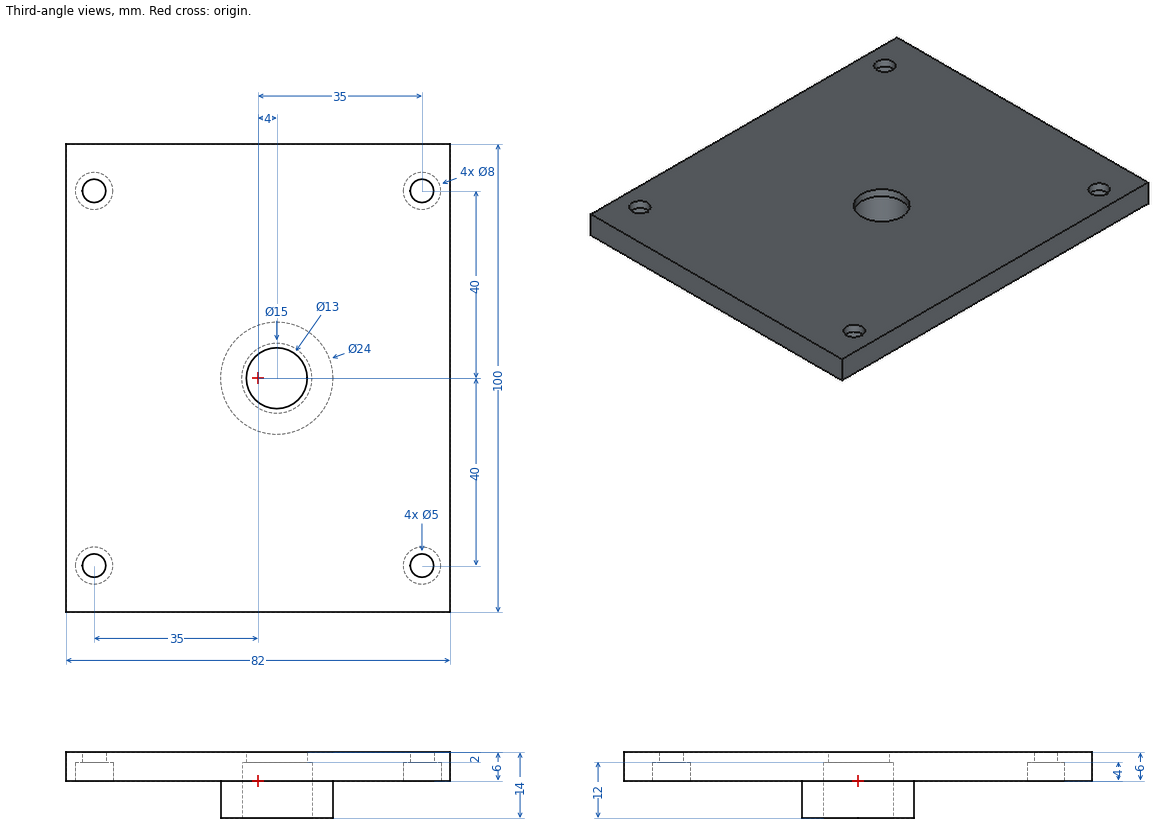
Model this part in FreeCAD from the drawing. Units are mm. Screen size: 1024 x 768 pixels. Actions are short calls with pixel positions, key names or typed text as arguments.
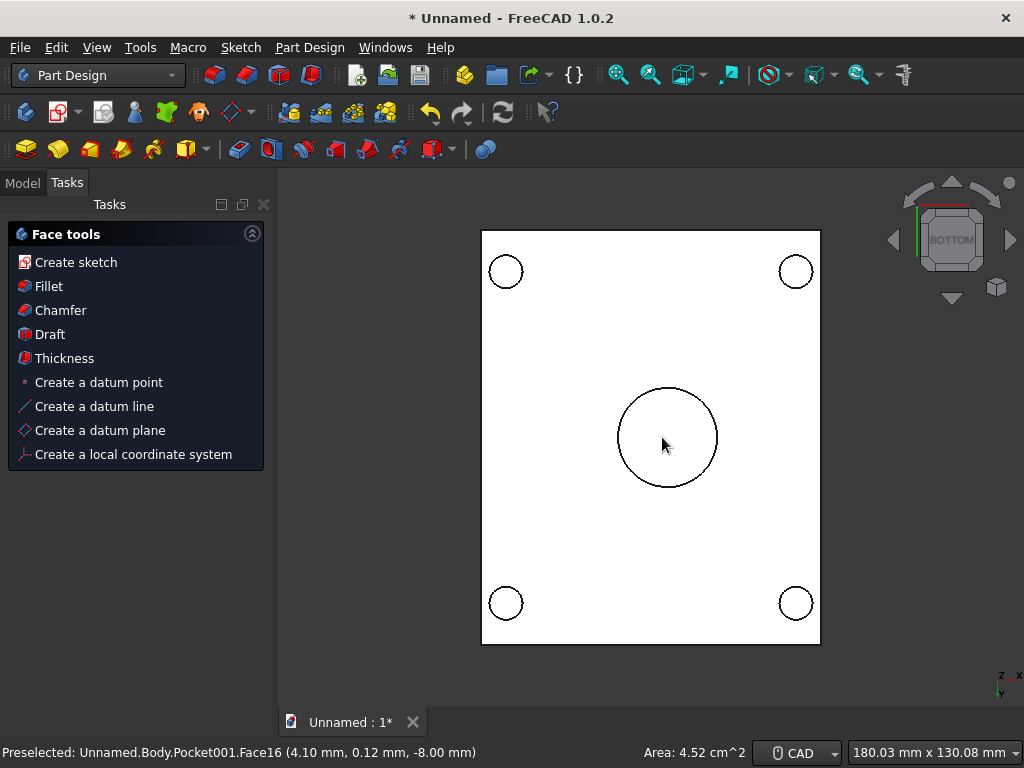
click(58, 112)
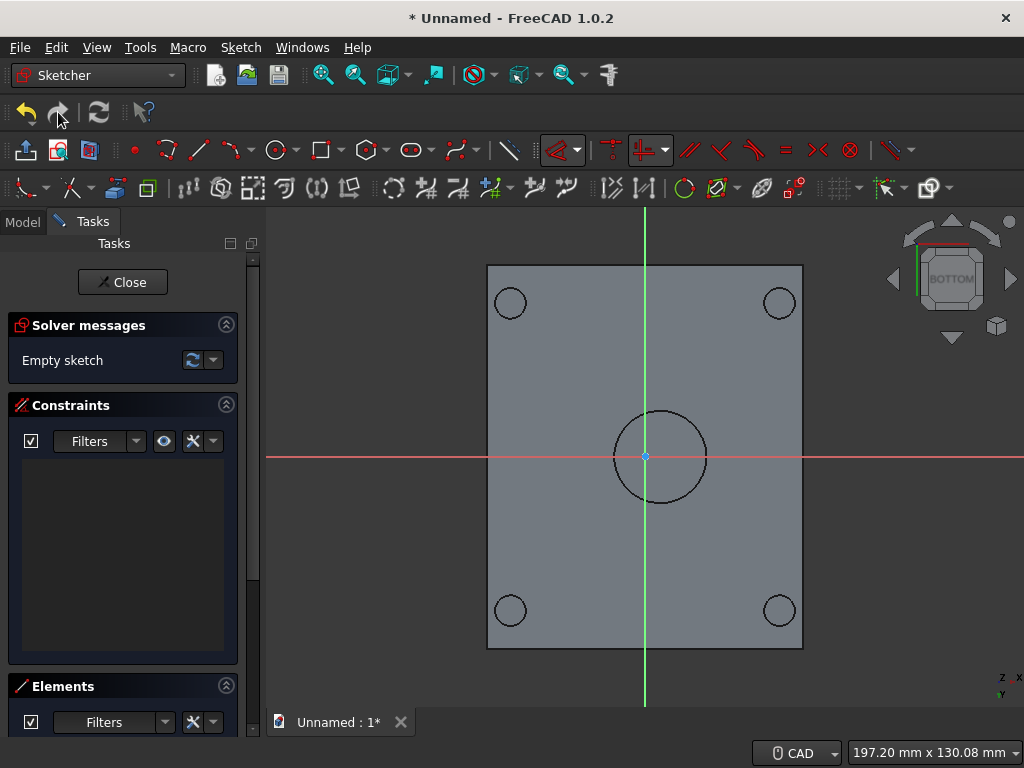
scroll(682, 457, up, 8)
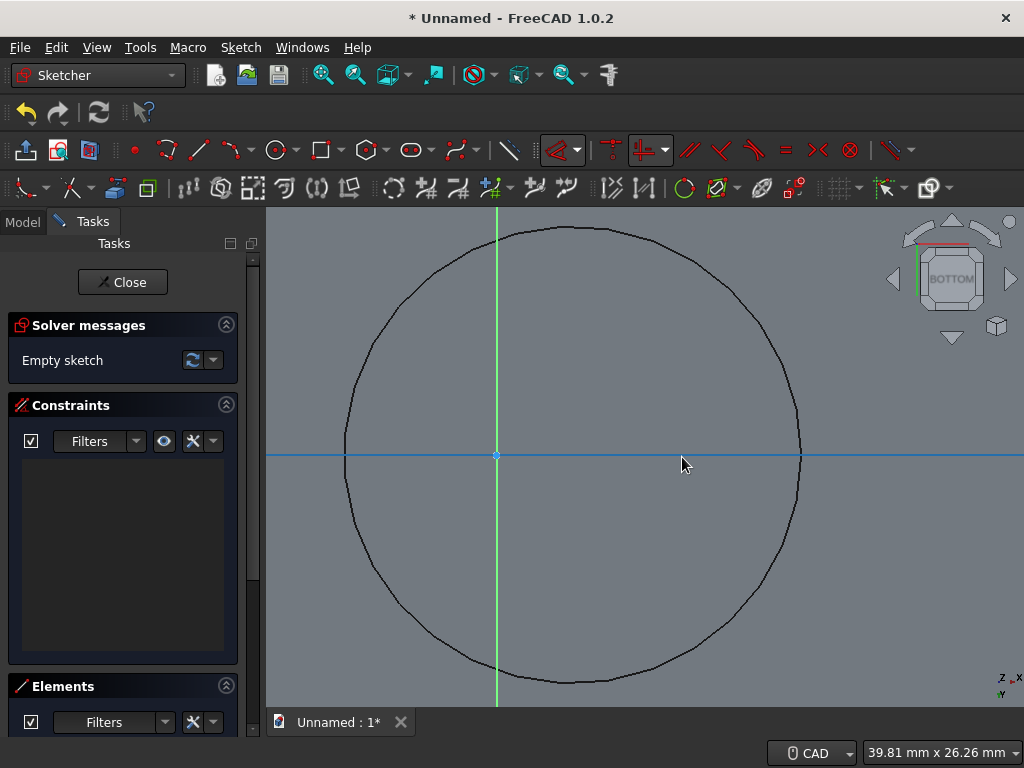
key(g)
key(c)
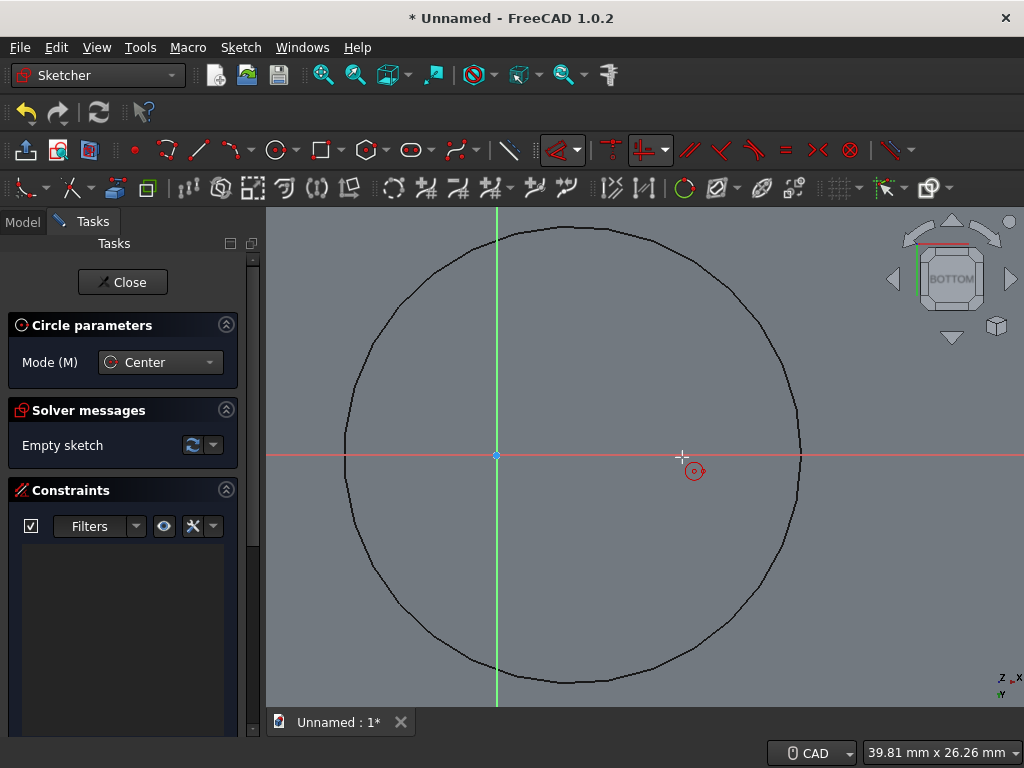
click(573, 455)
move(674, 354)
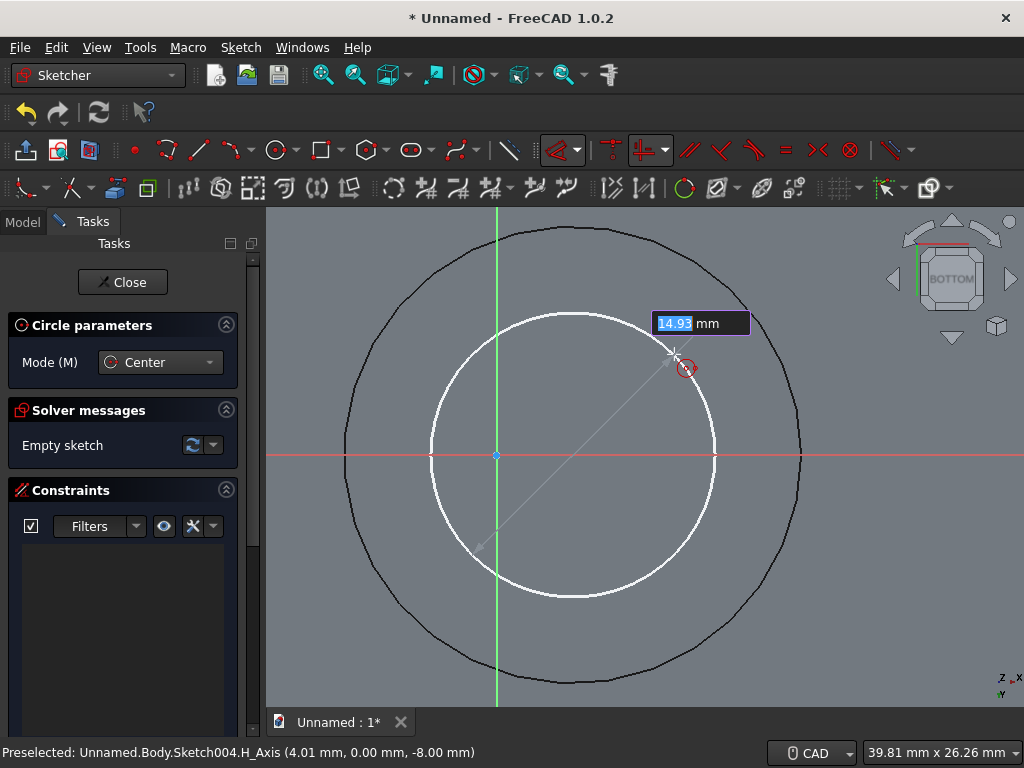
text(15)
key(Return)
key(Escape)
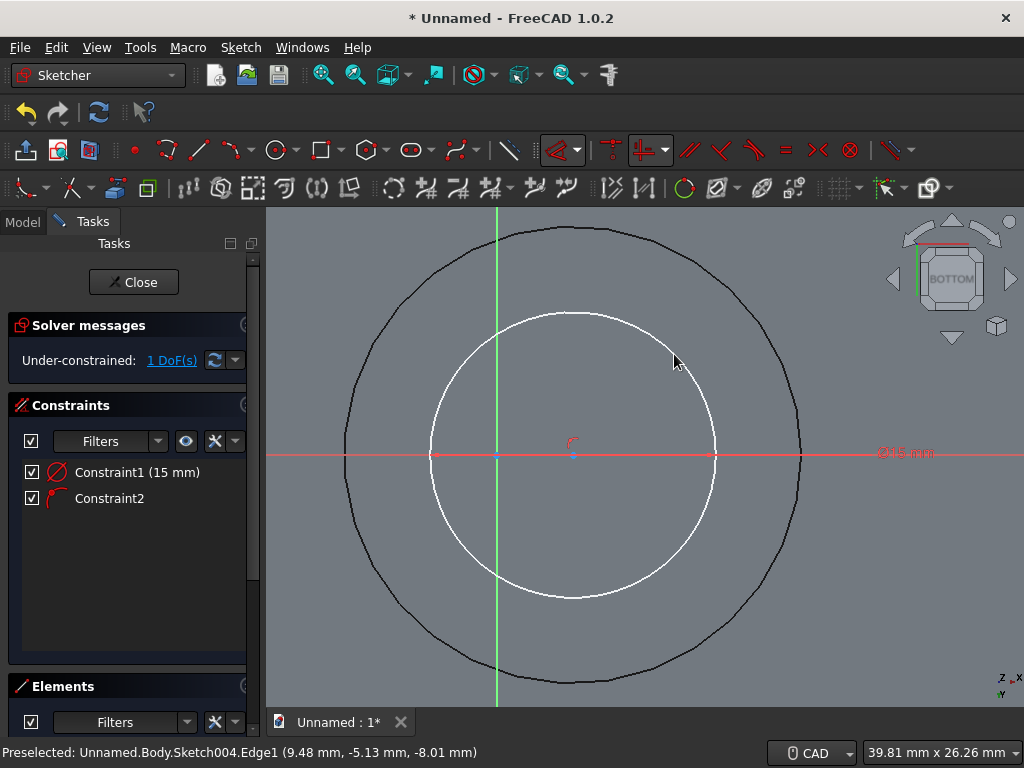
click(573, 455)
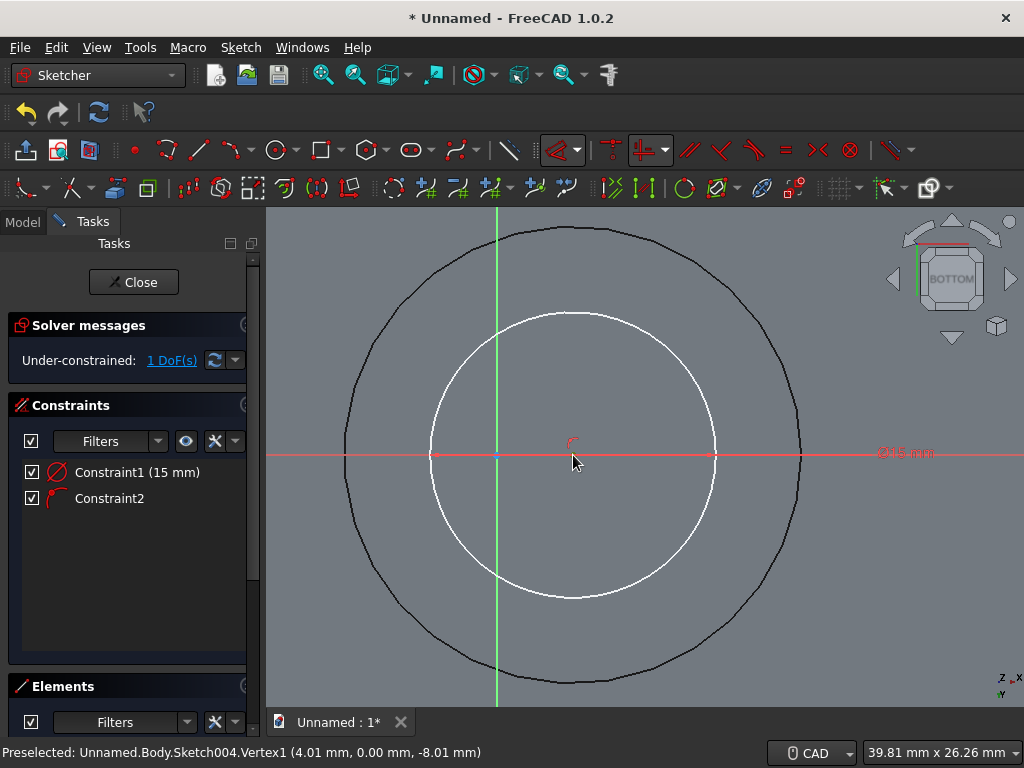
click(580, 150)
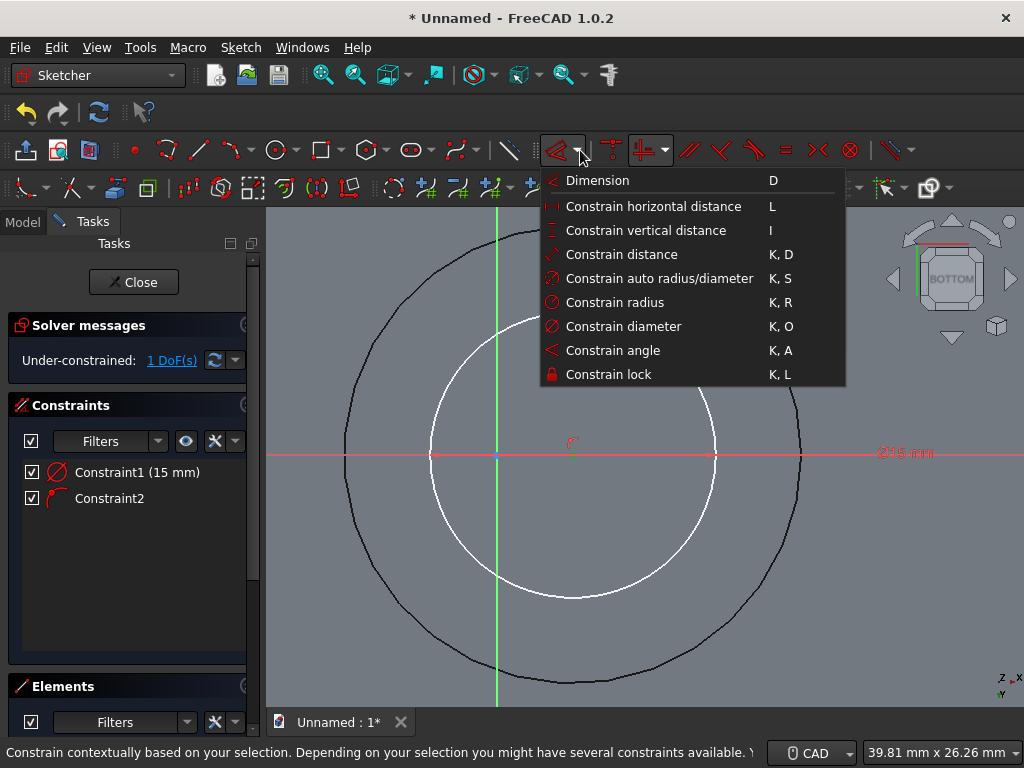
click(693, 206)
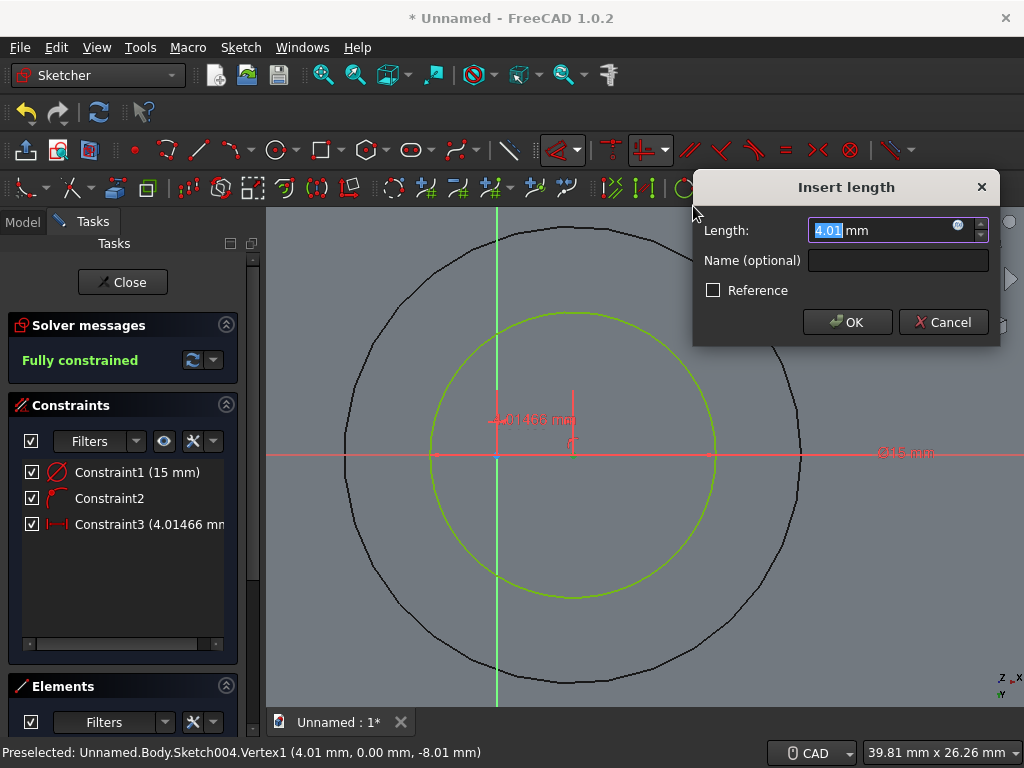
text(4)
key(Return)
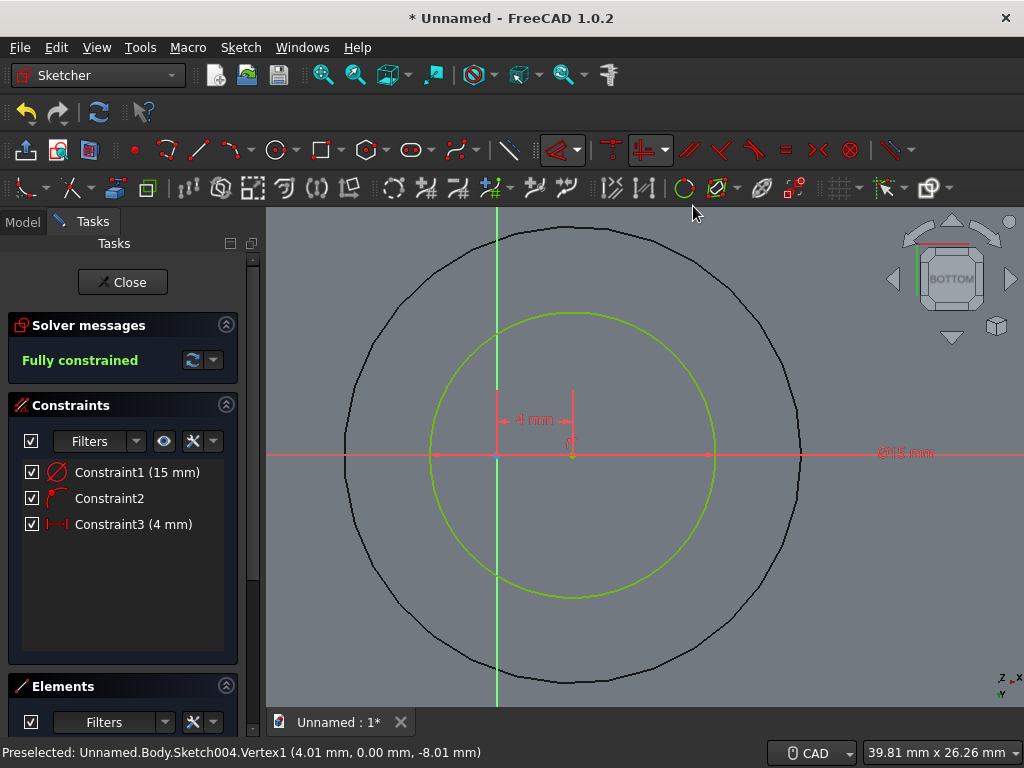
click(123, 282)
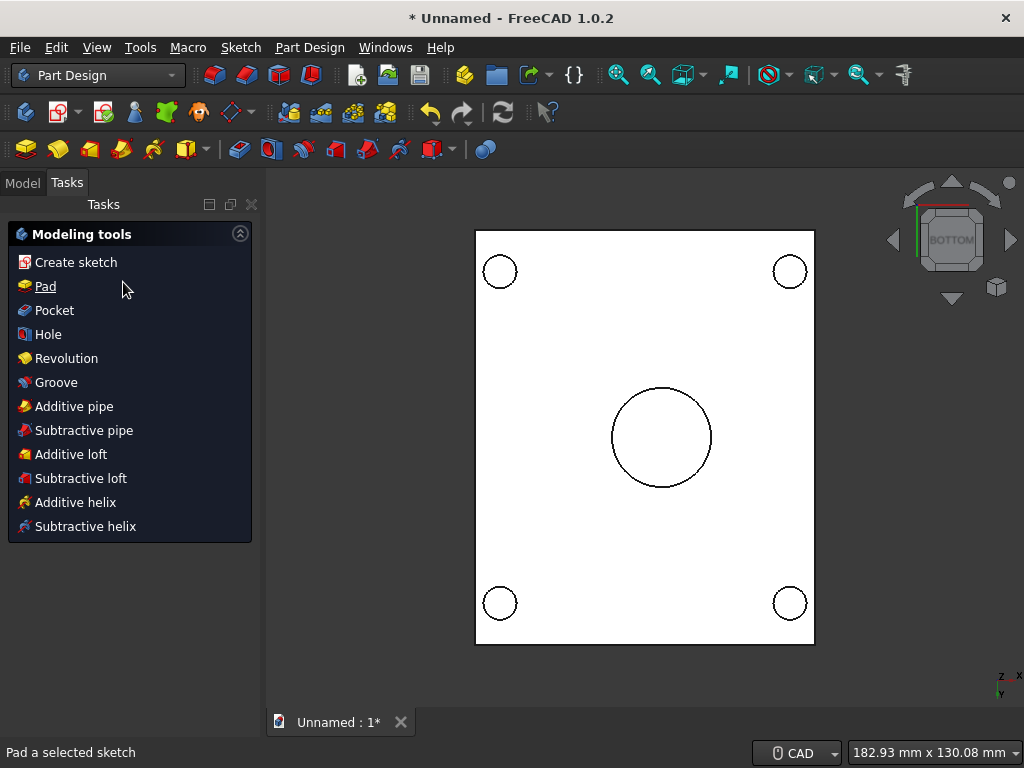
click(240, 150)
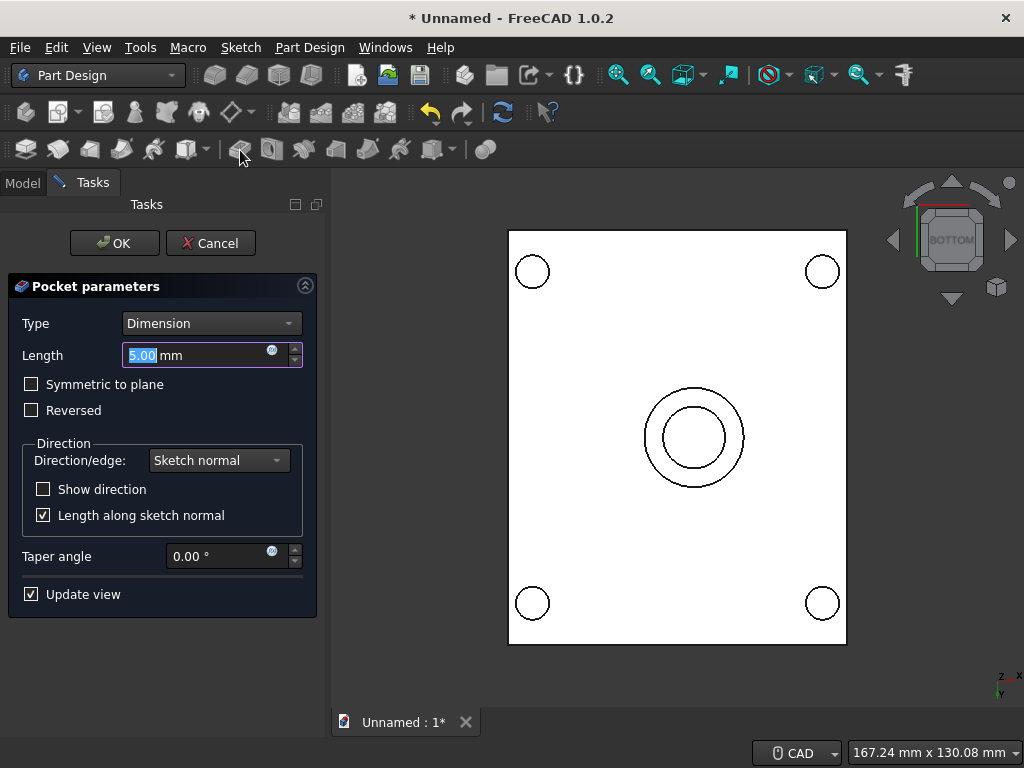
text(12)
key(Tab)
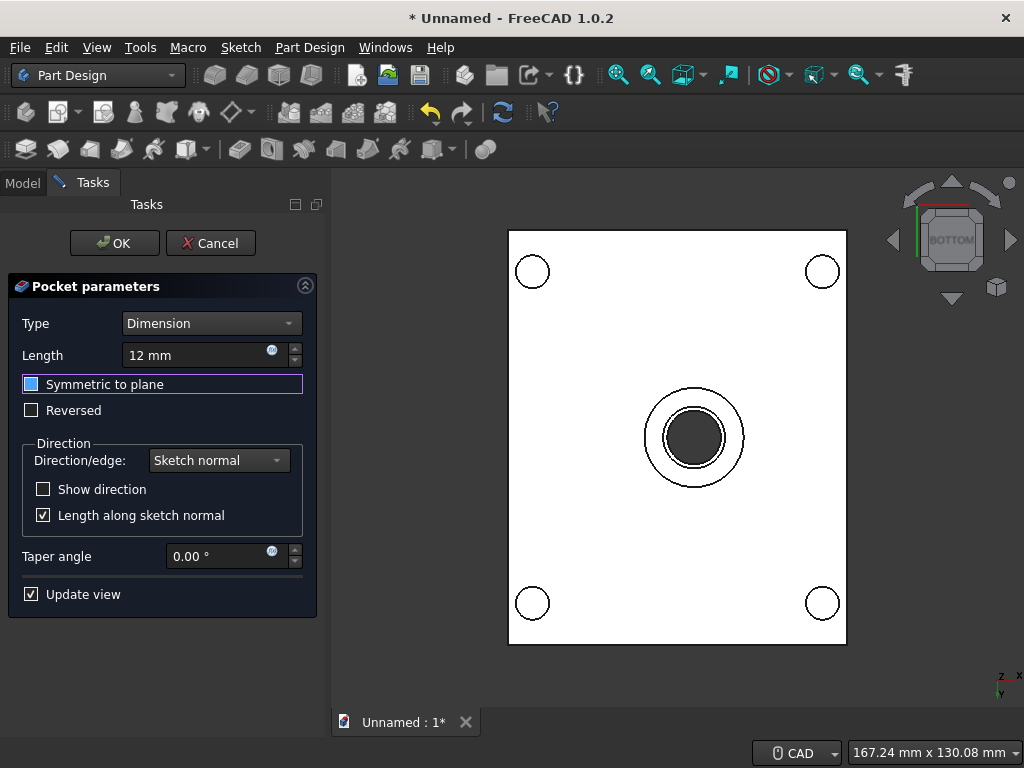
click(115, 243)